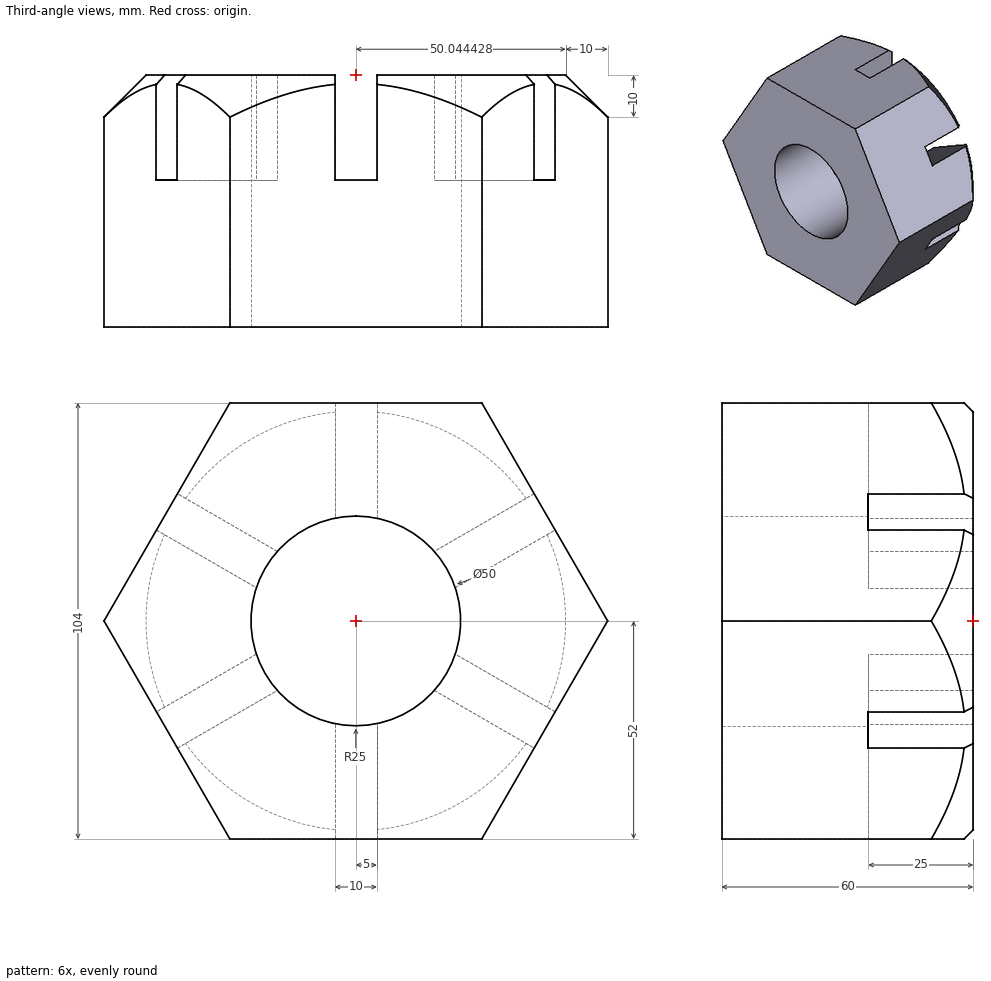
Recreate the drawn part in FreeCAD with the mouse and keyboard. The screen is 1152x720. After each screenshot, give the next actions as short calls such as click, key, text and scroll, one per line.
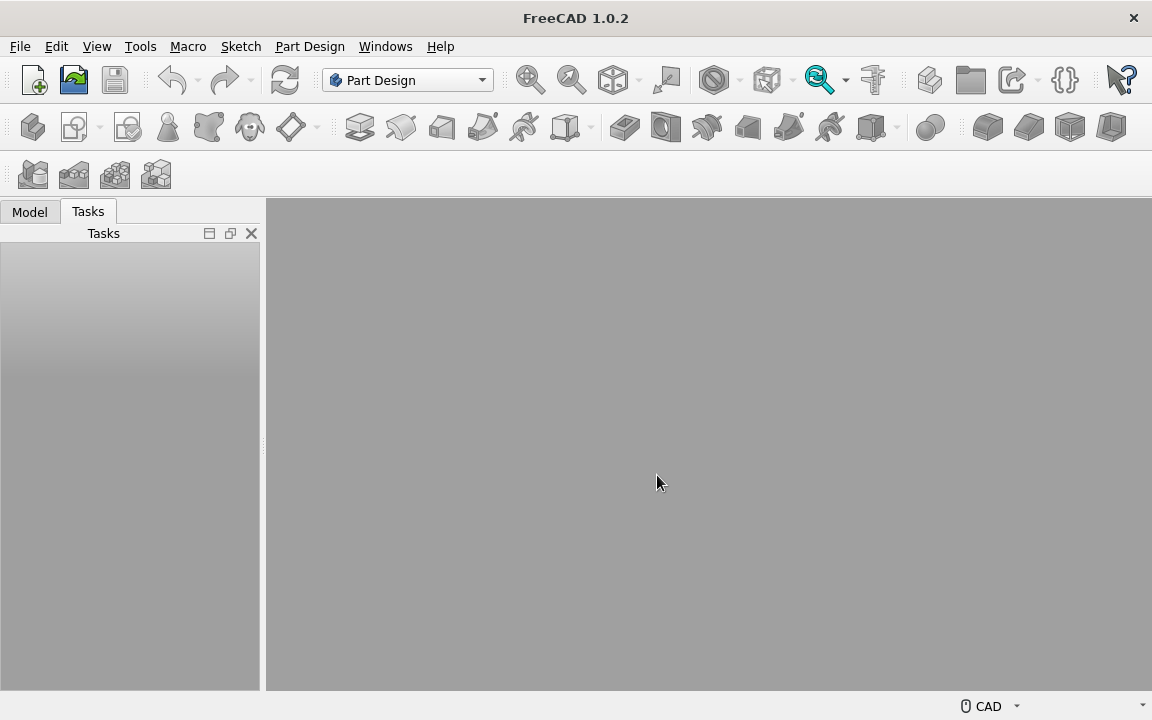
click(33, 80)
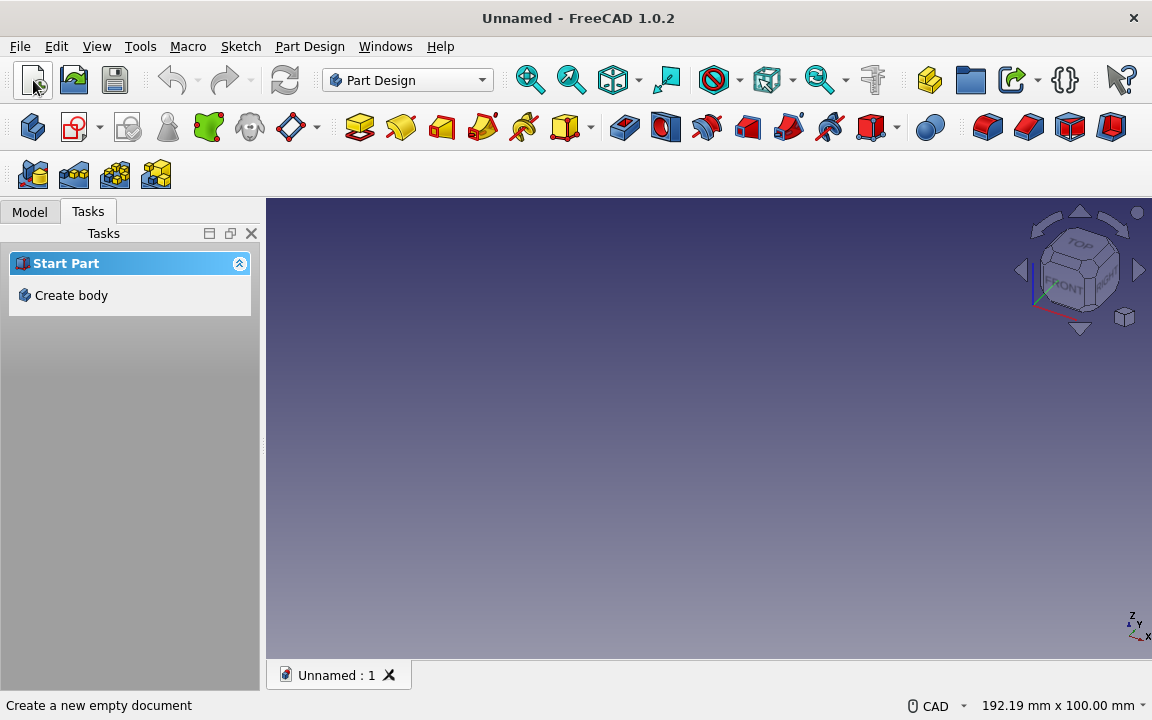
click(74, 128)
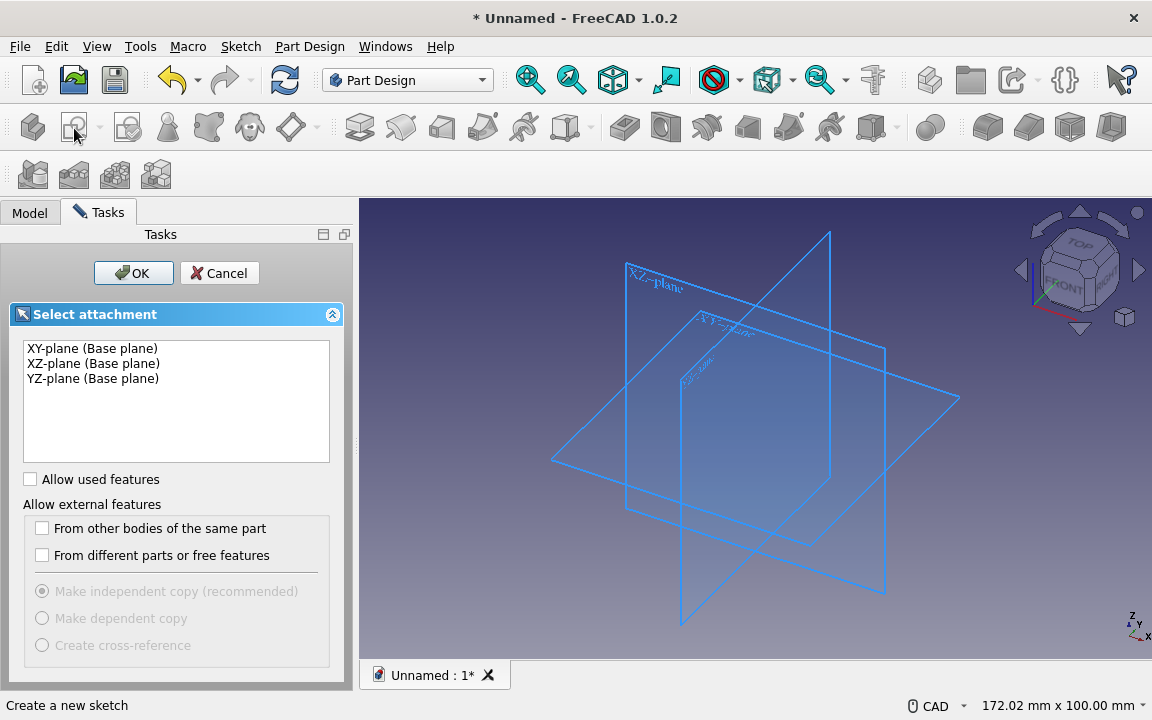
click(84, 364)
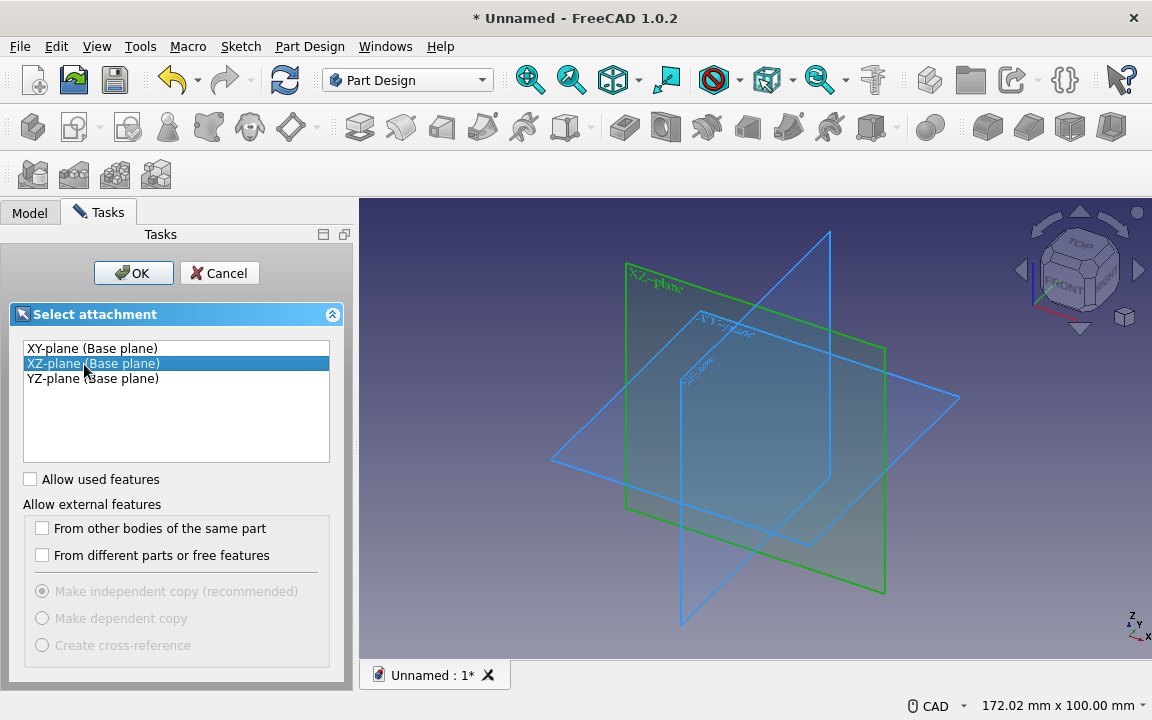
click(134, 273)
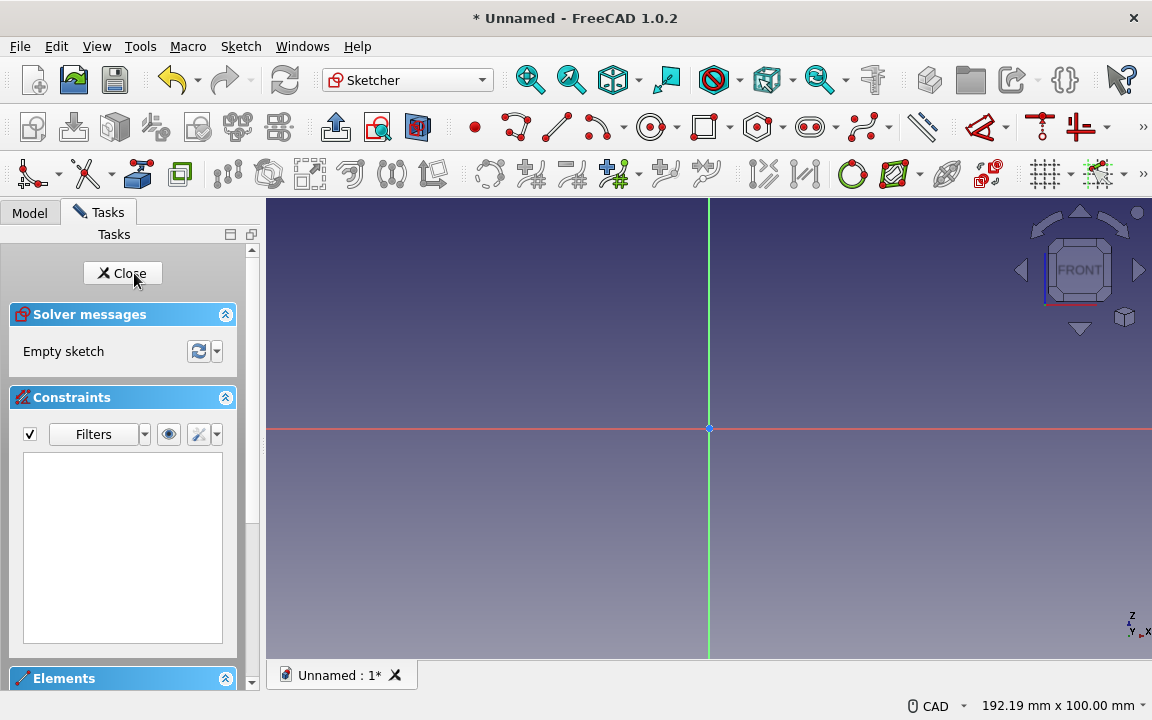
scroll(557, 428, down, 3)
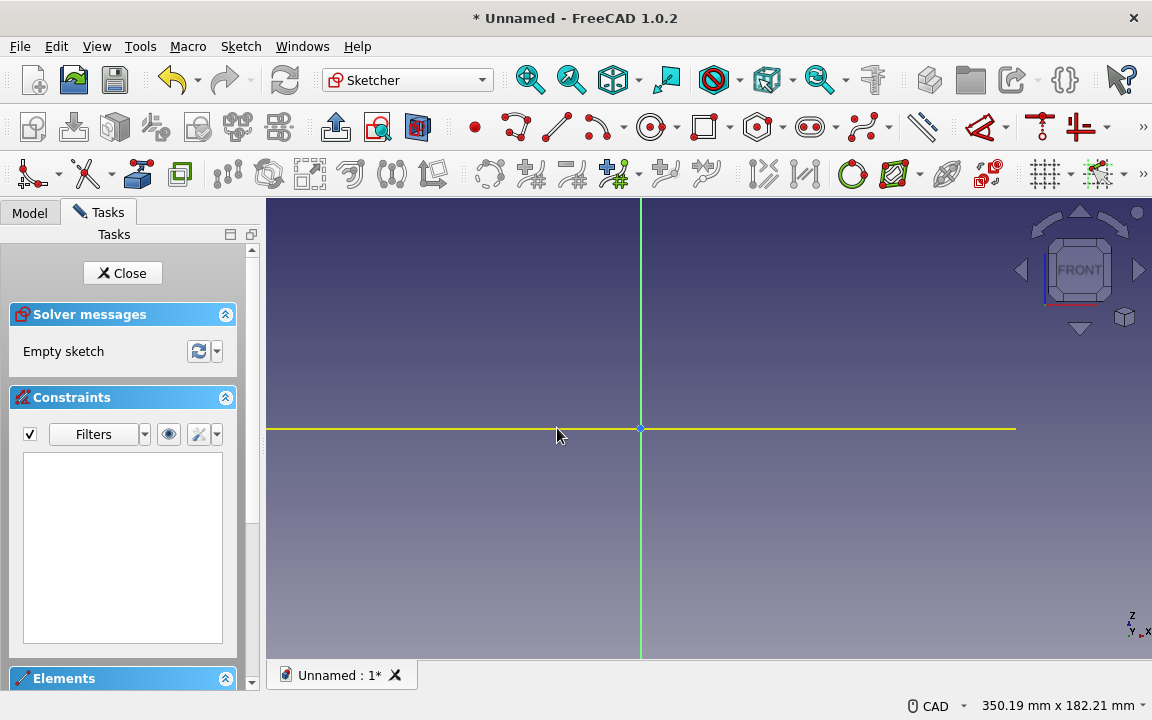
click(756, 128)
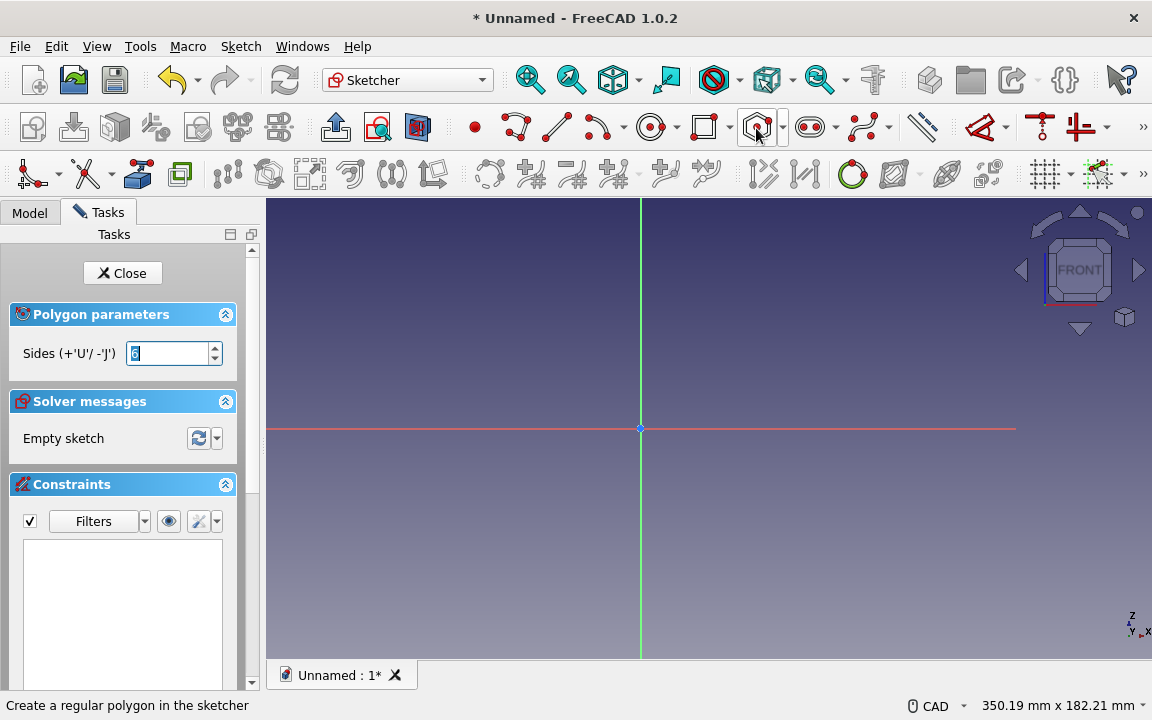
click(641, 428)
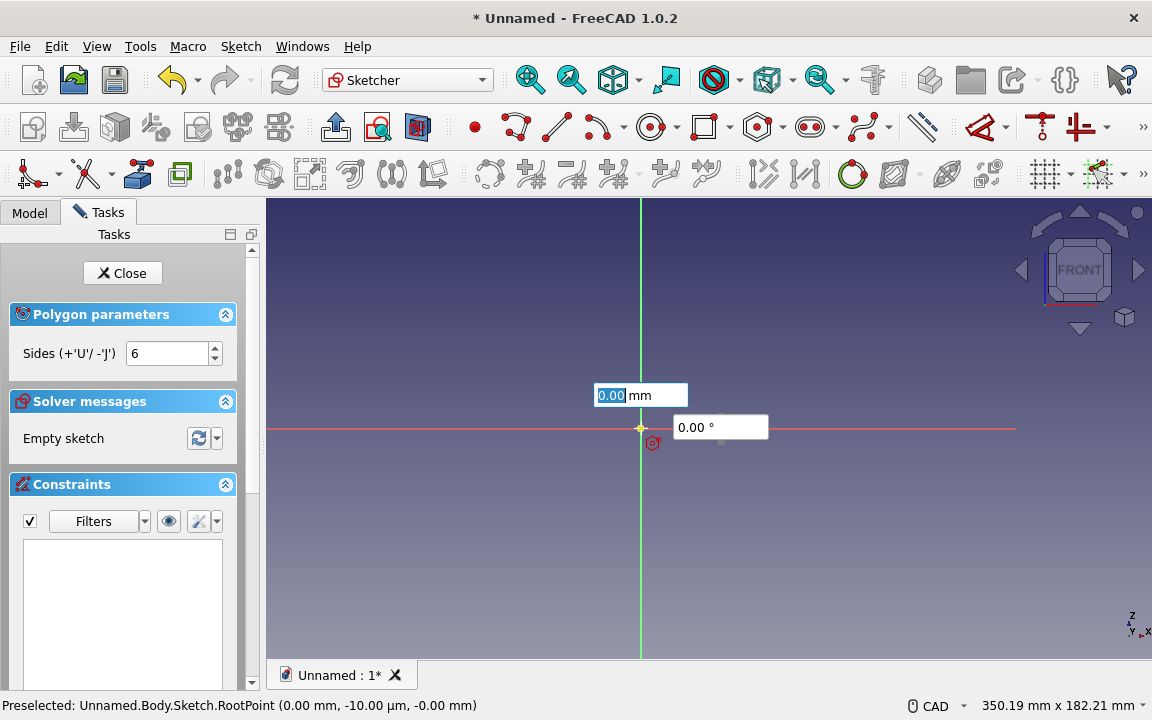
click(792, 428)
right_click(792, 428)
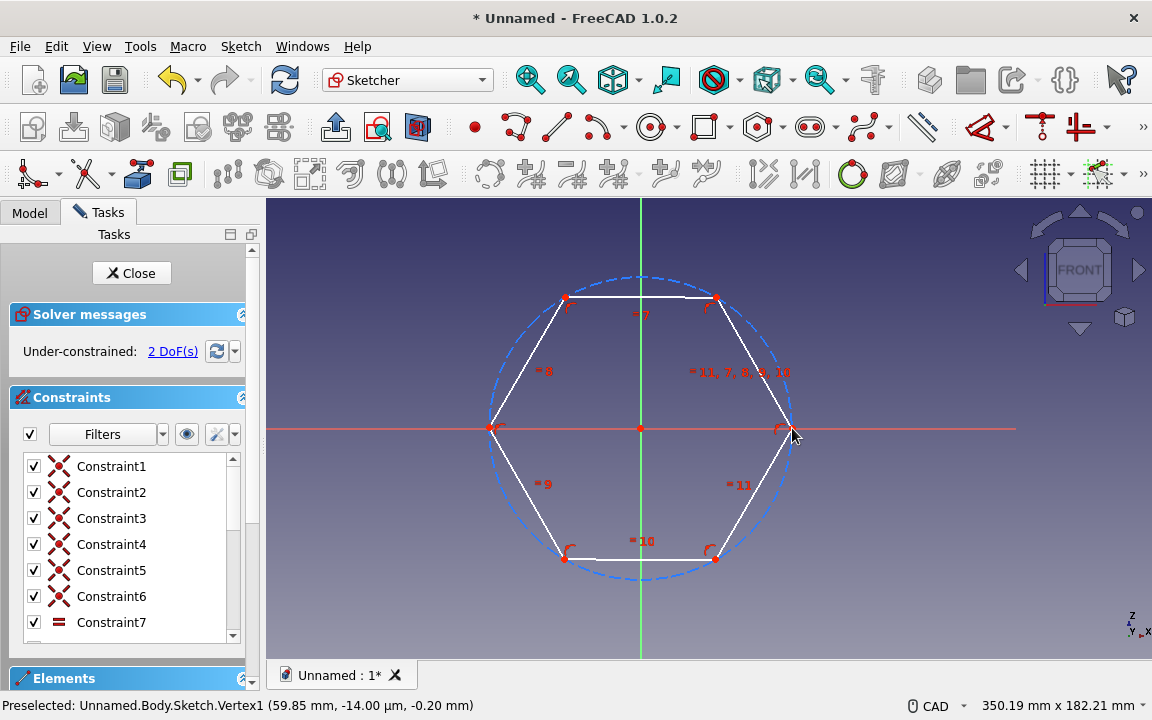
click(650, 128)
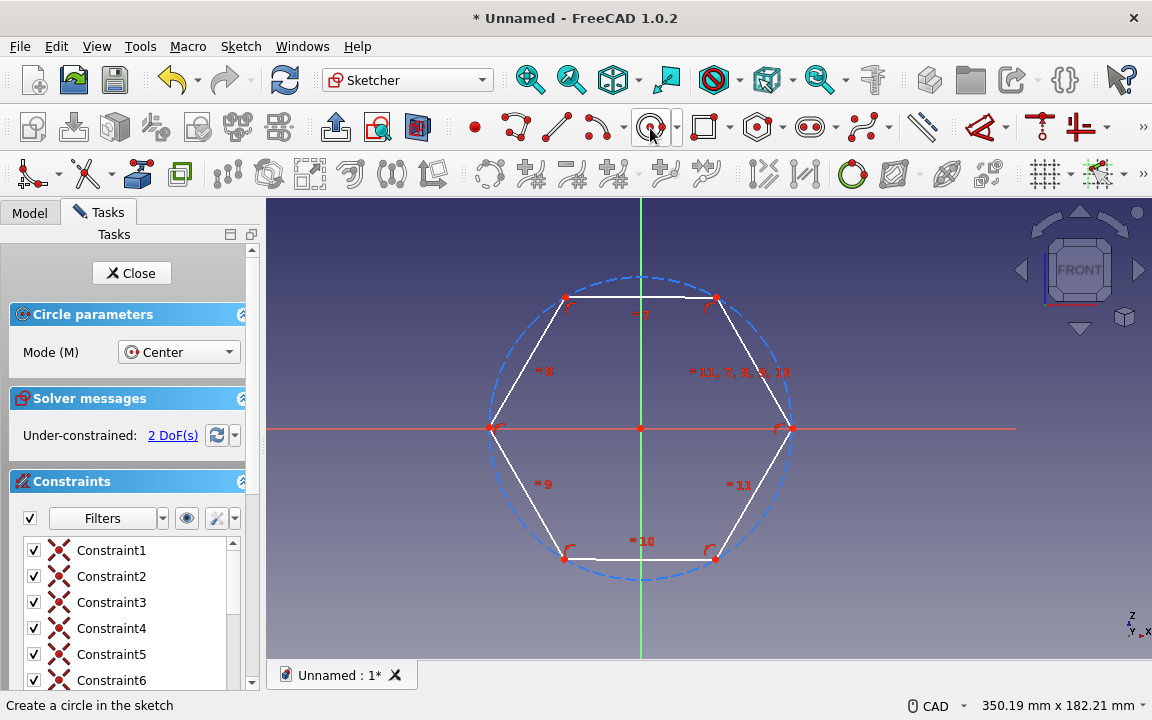
click(641, 428)
move(685, 384)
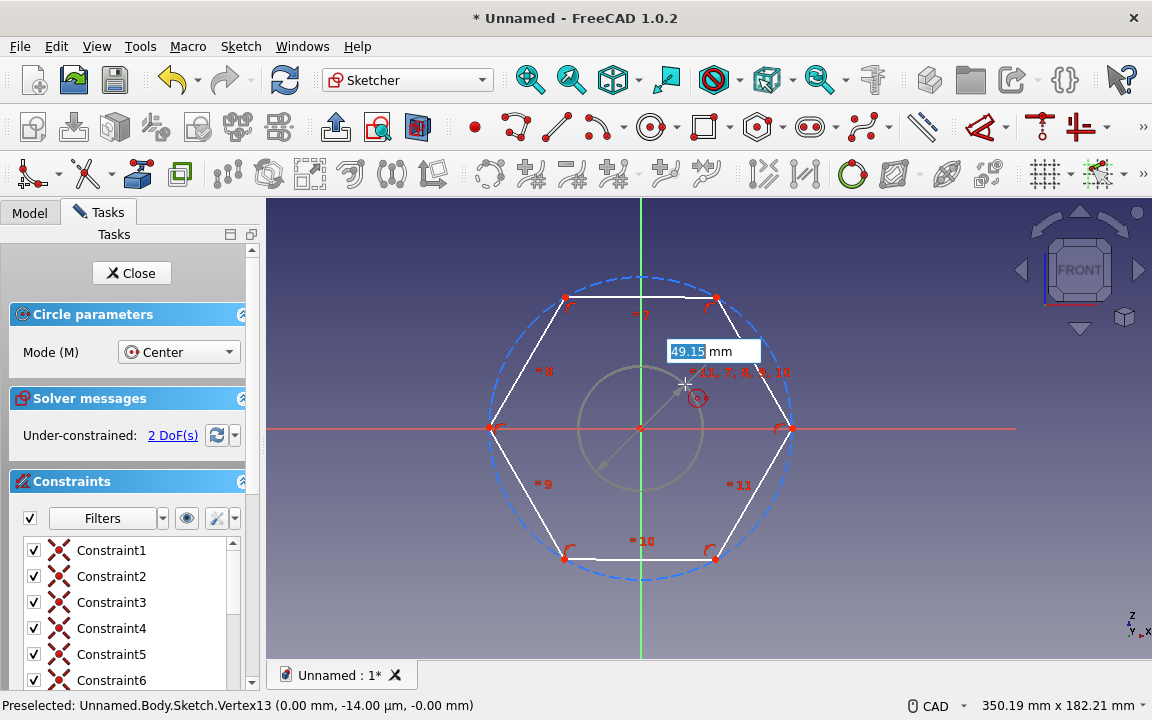
text(50)
key(Return)
key(Escape)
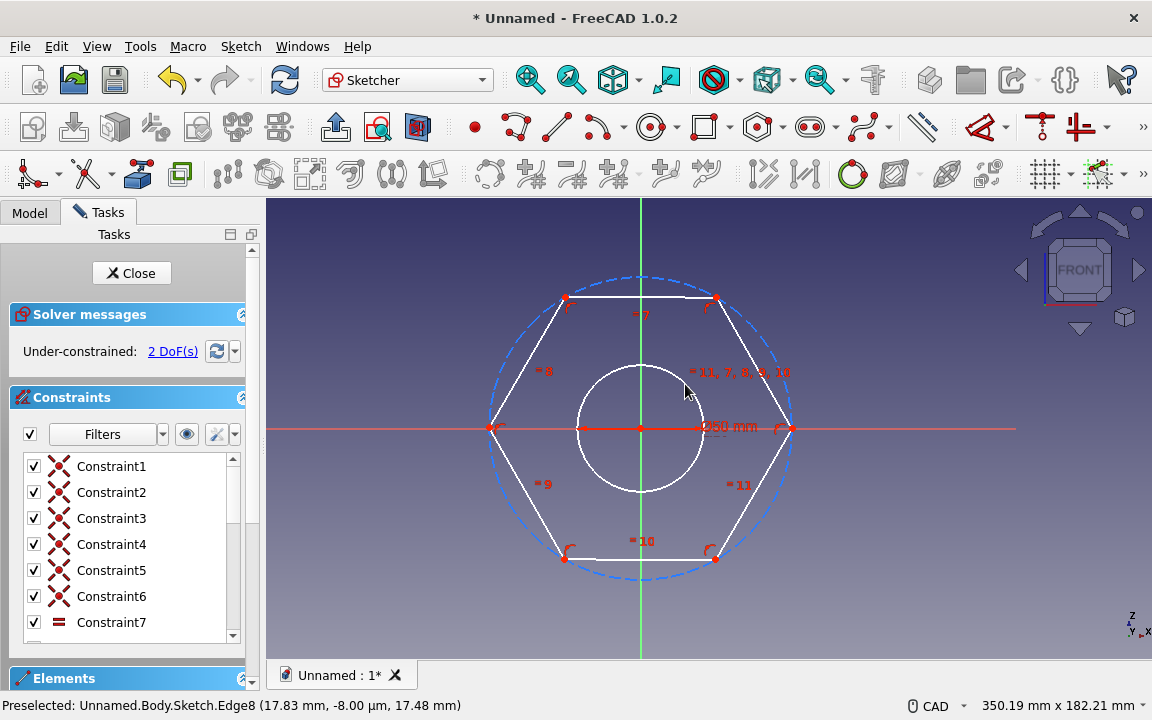
click(671, 297)